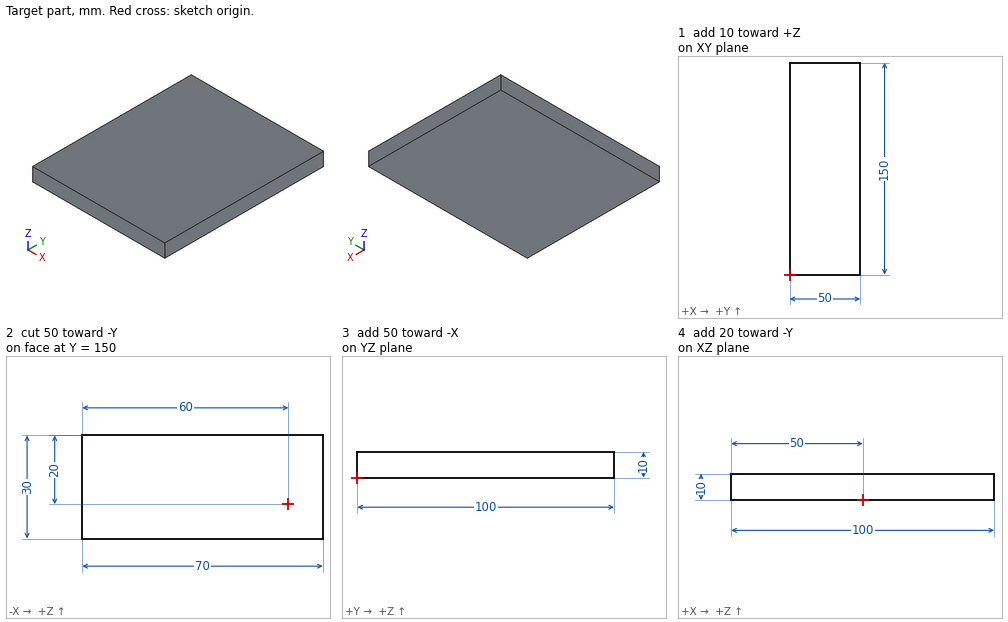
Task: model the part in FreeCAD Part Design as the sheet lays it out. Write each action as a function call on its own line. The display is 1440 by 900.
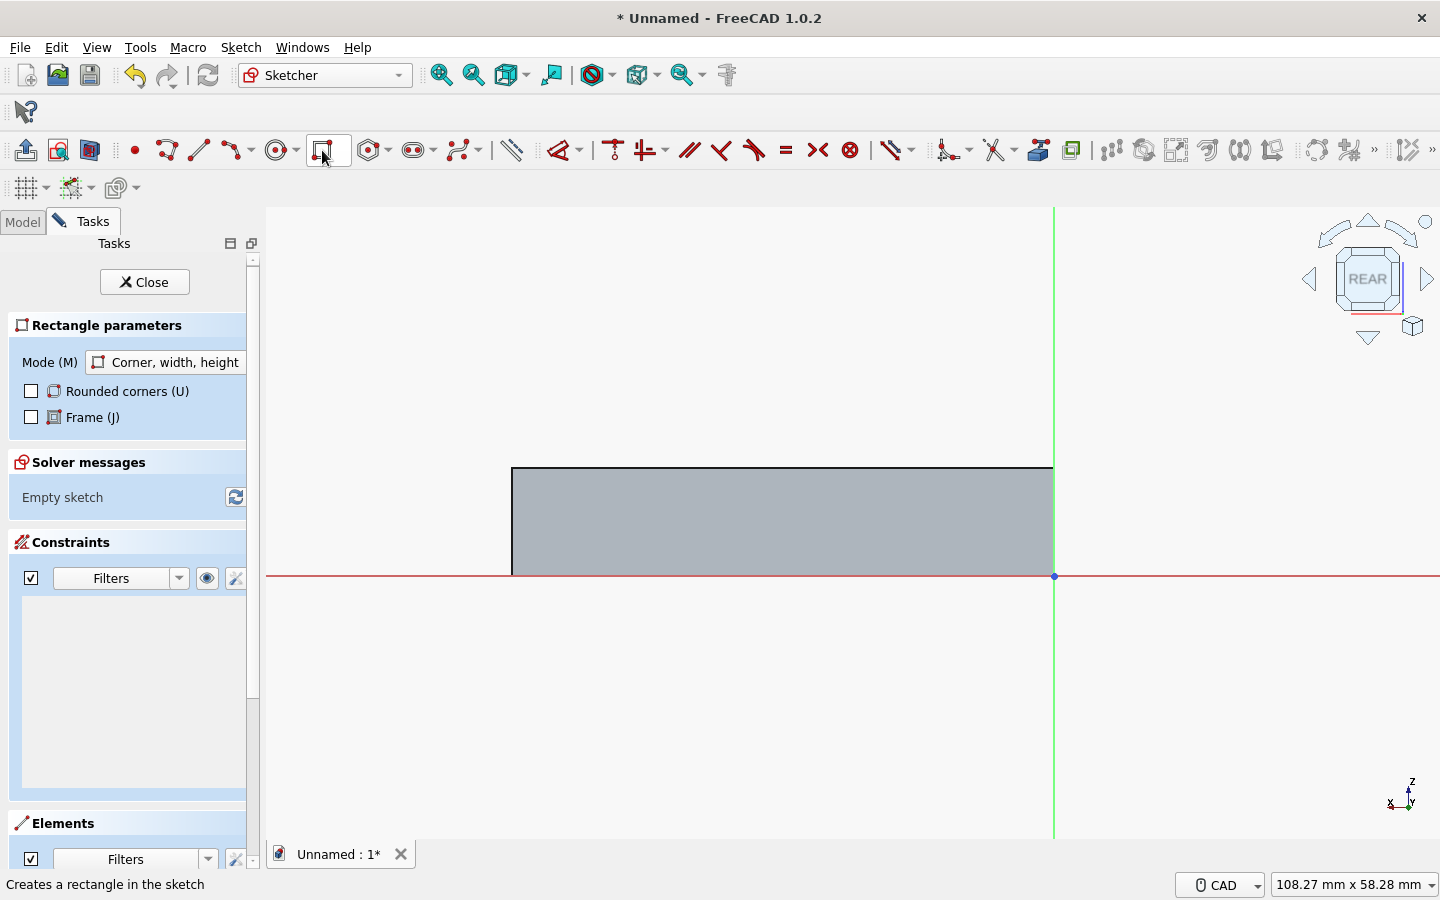
click(404, 359)
click(1163, 685)
key(Escape)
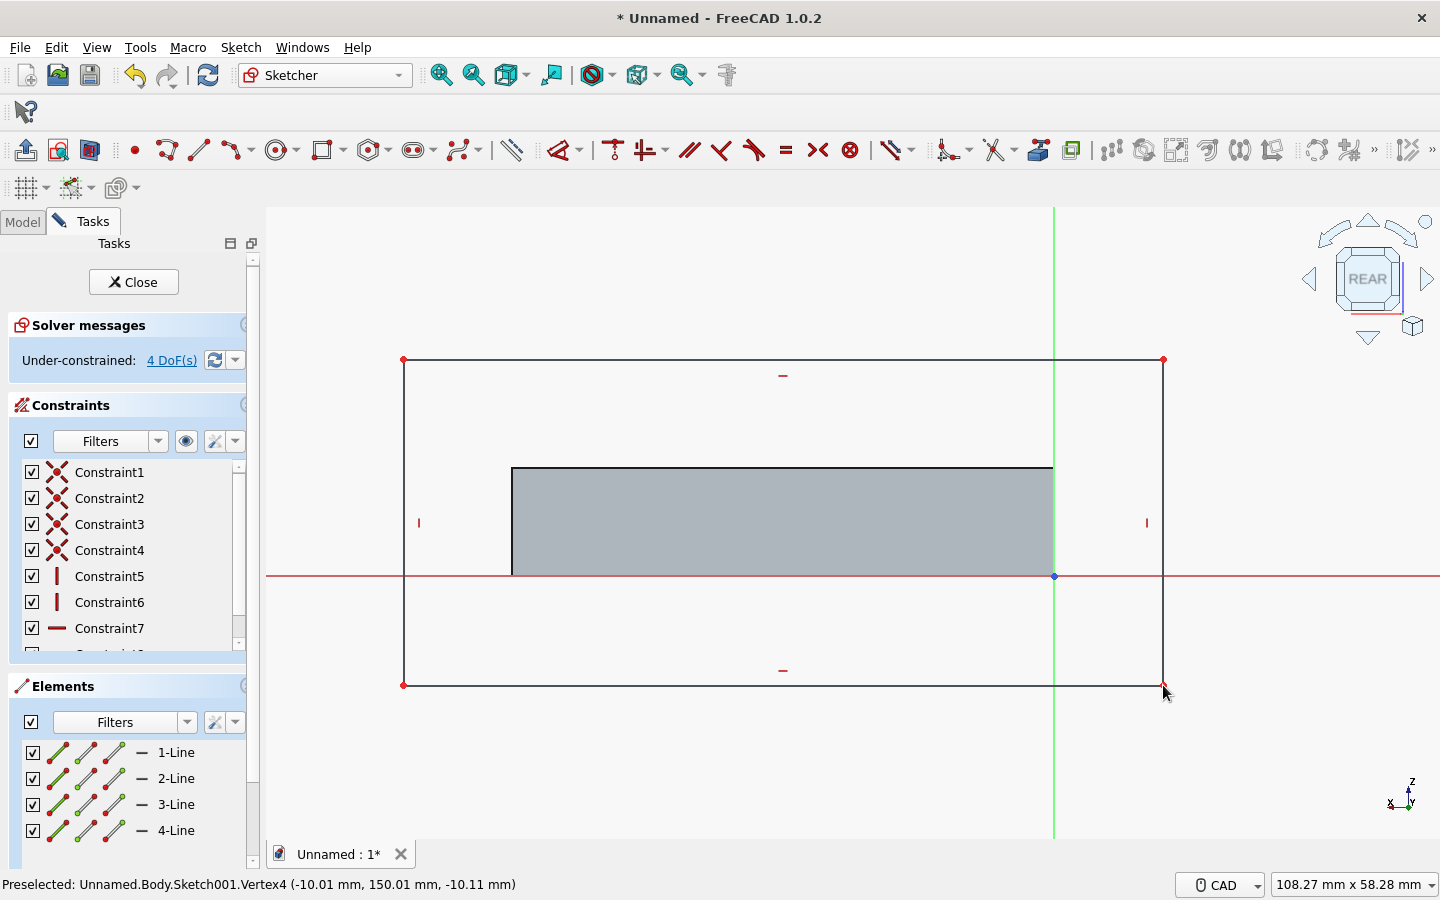
click(558, 150)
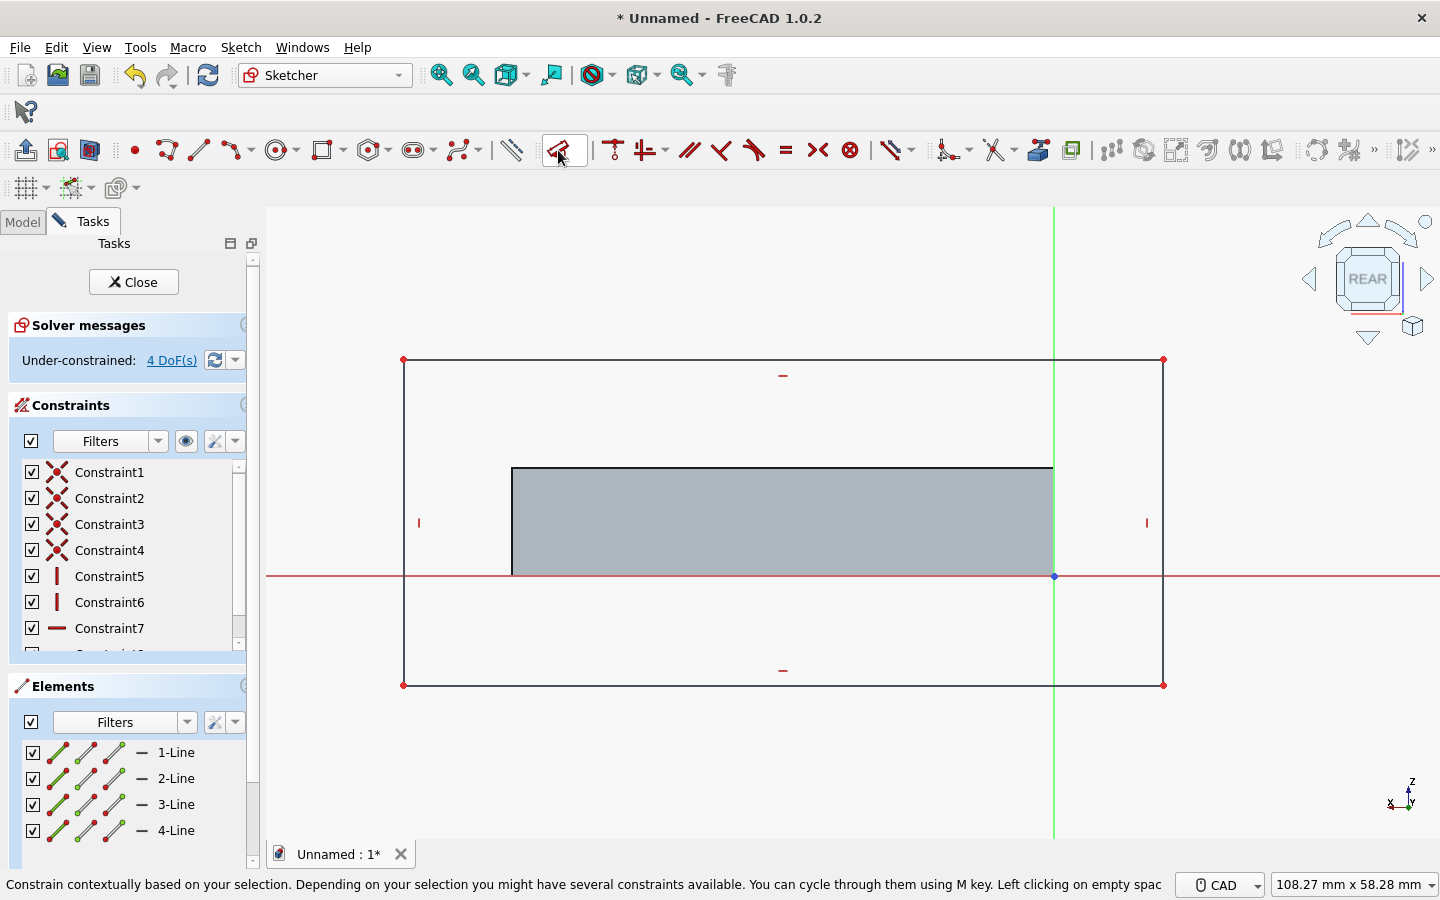
click(404, 458)
click(370, 523)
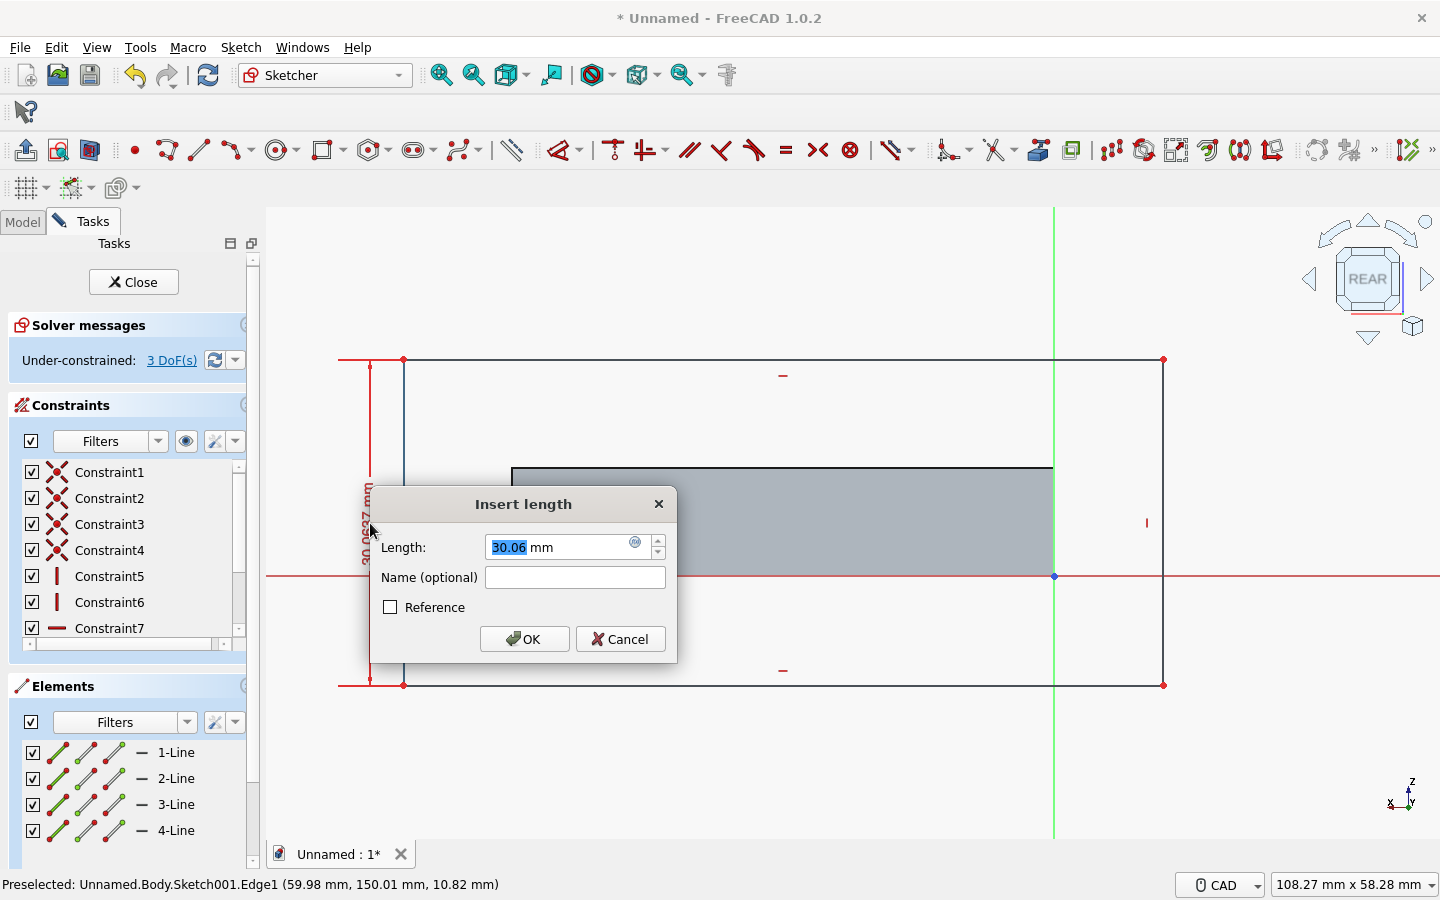
text(30)
key(Return)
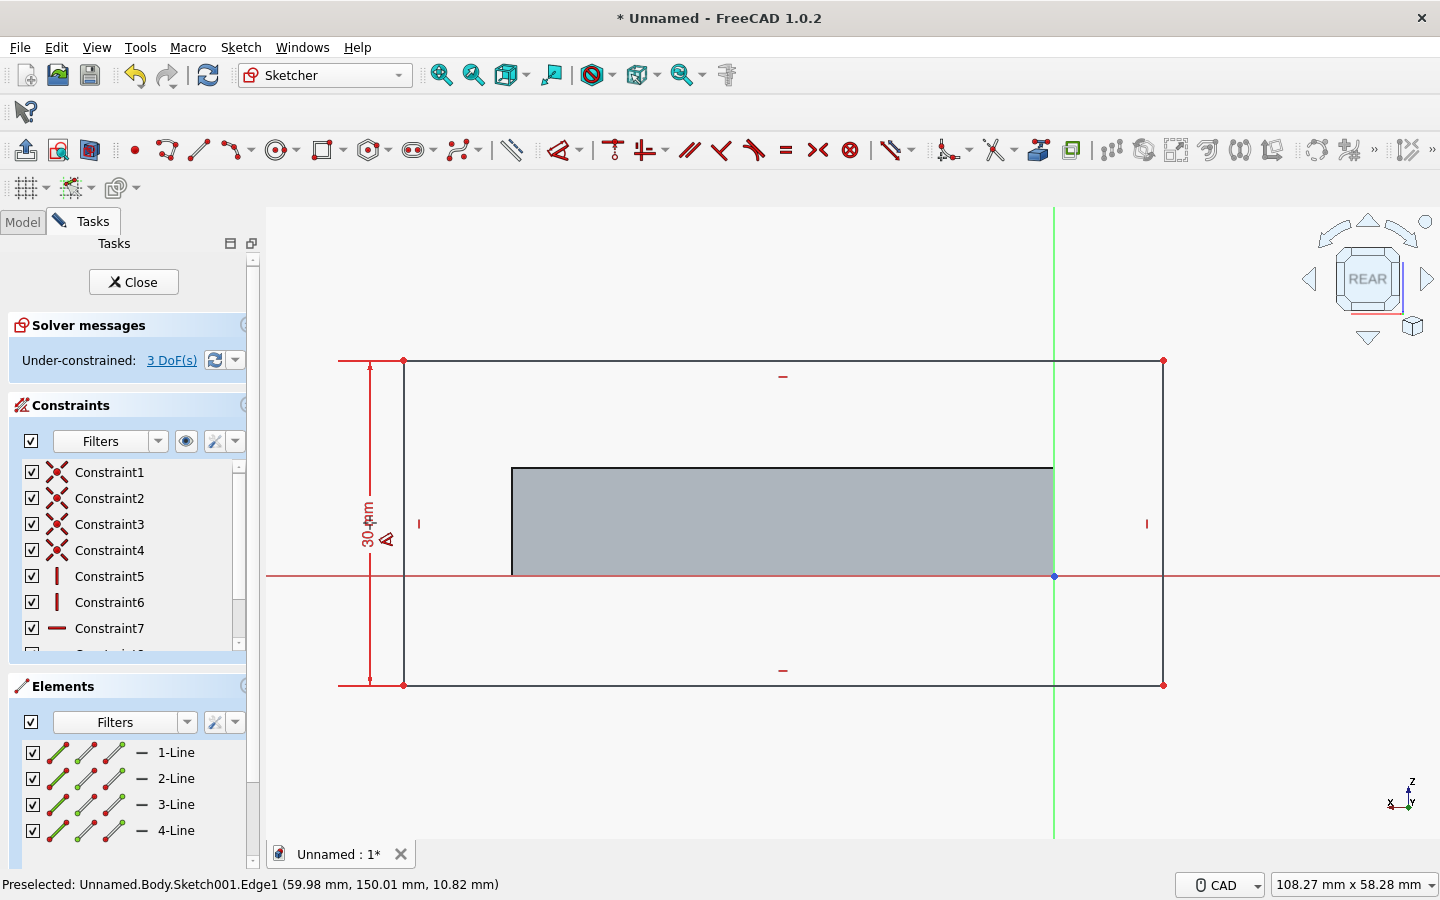
click(632, 686)
click(784, 720)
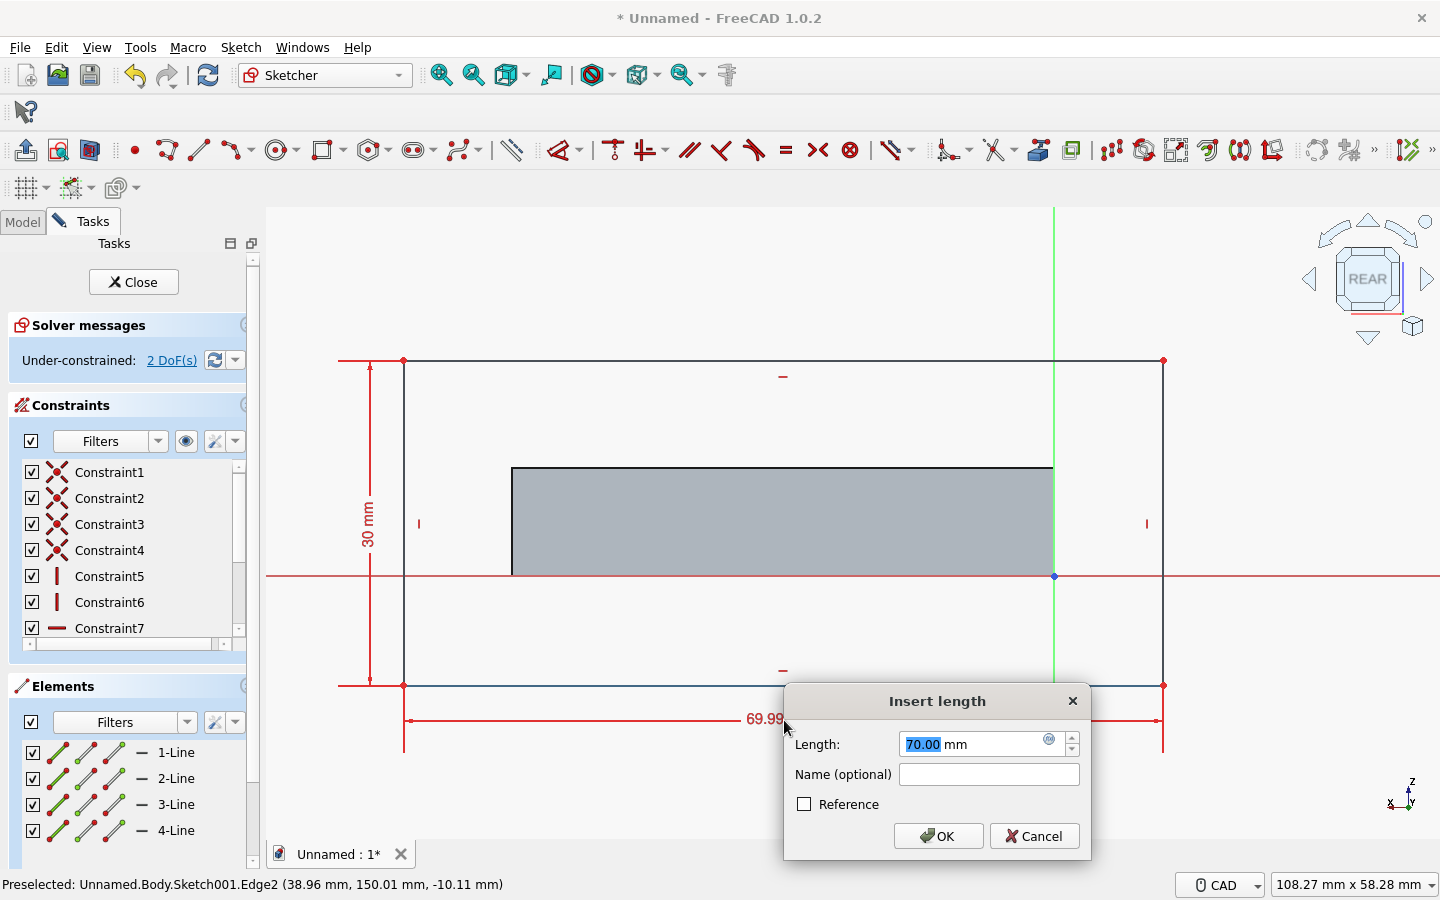
text(70)
key(Return)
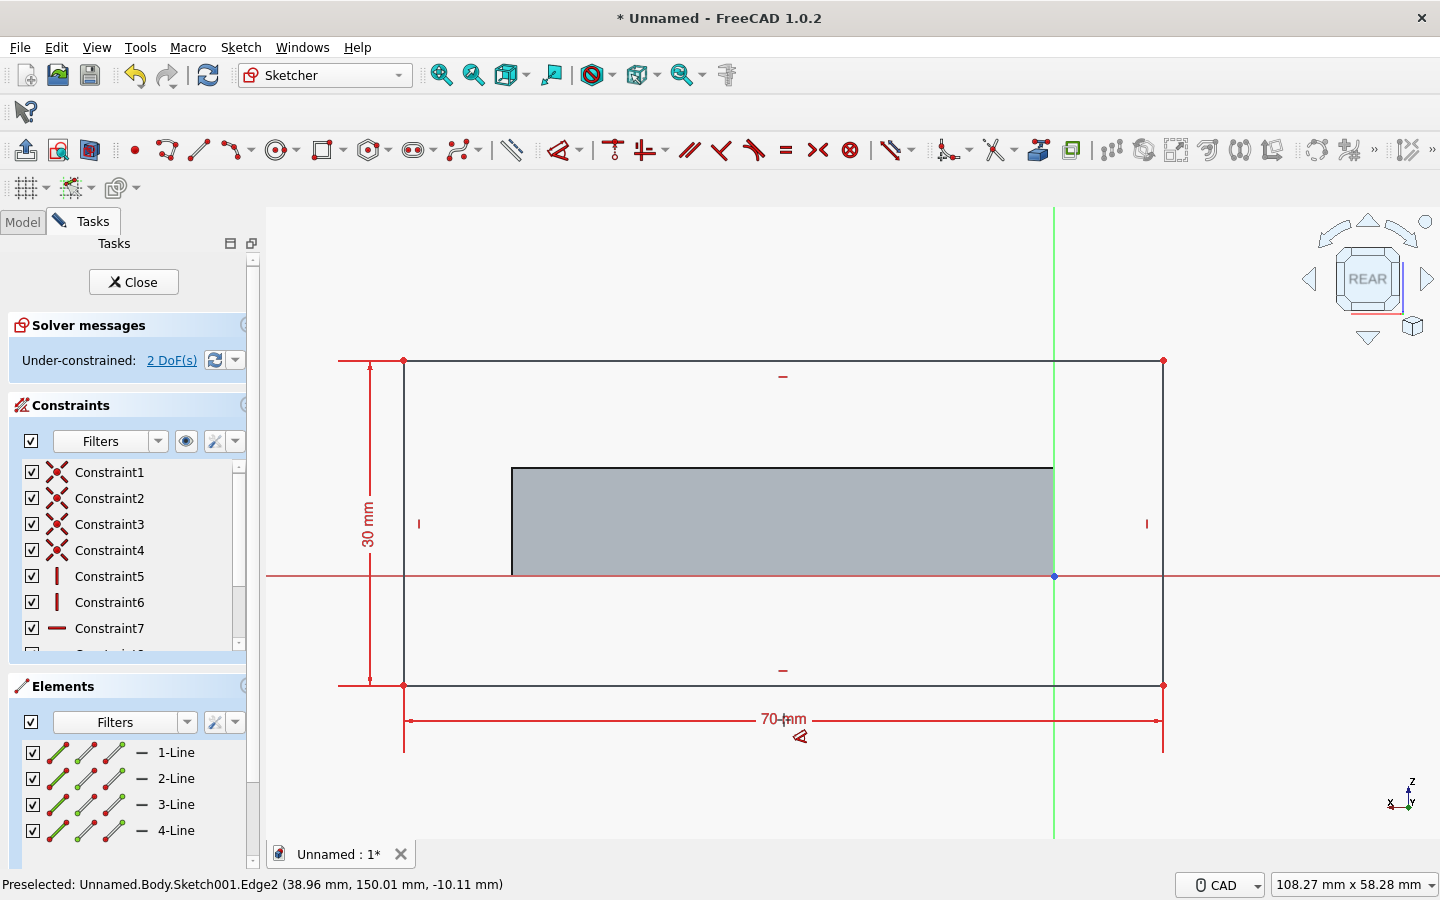
click(404, 361)
click(729, 327)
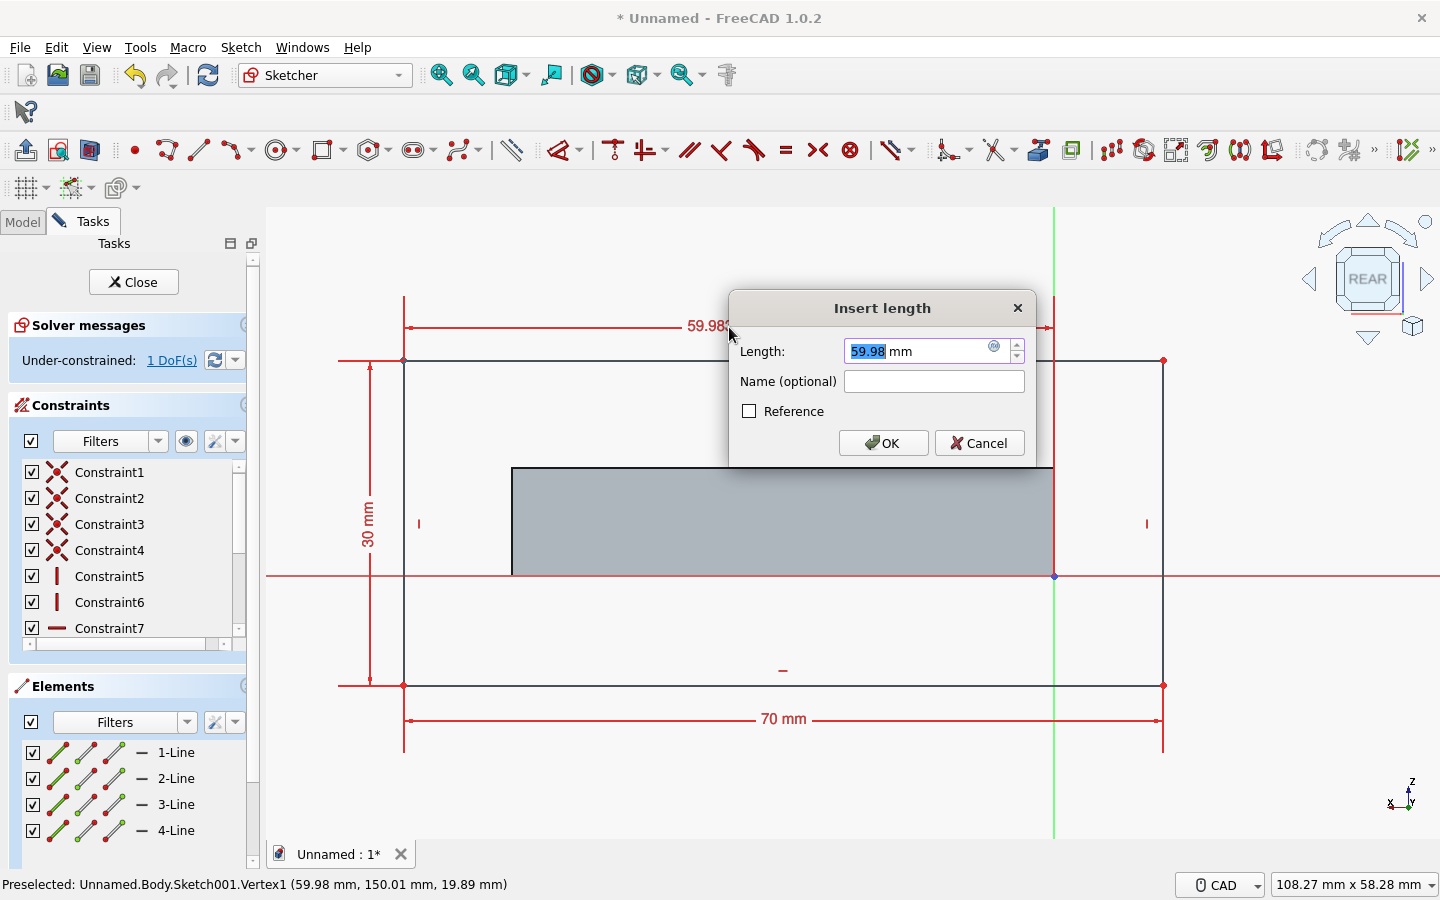
text(60)
key(Return)